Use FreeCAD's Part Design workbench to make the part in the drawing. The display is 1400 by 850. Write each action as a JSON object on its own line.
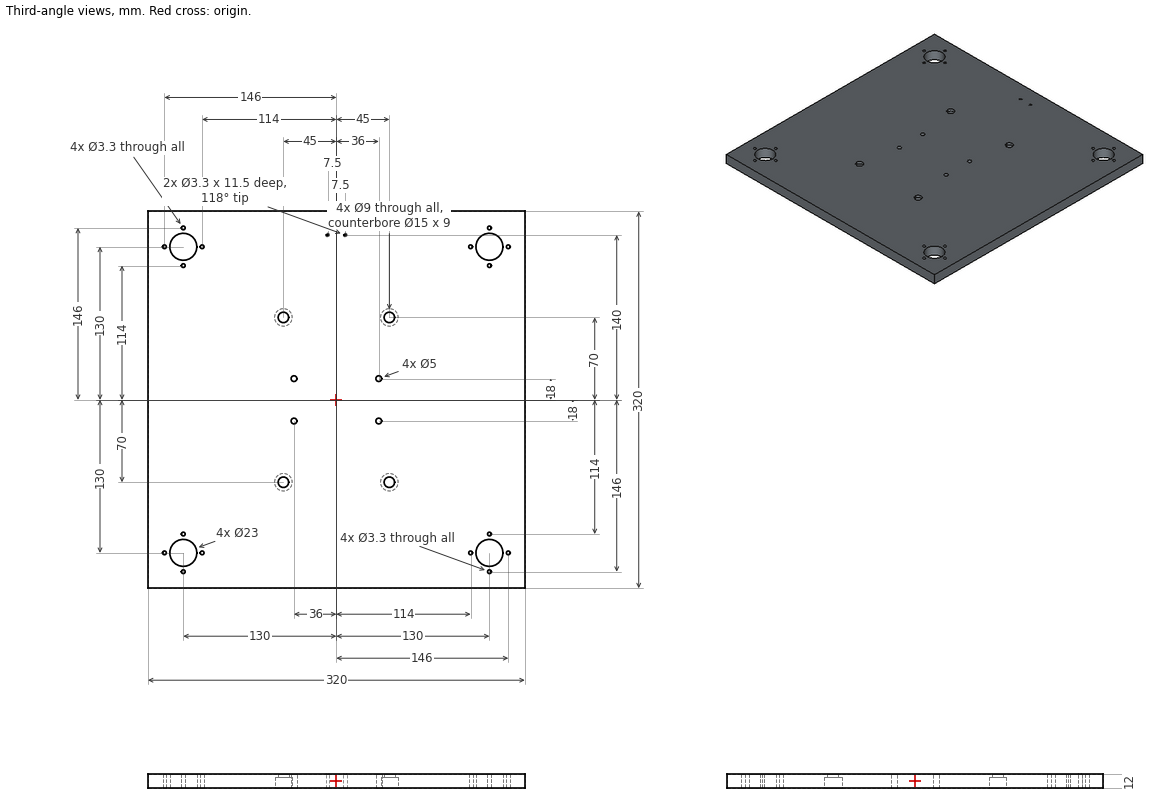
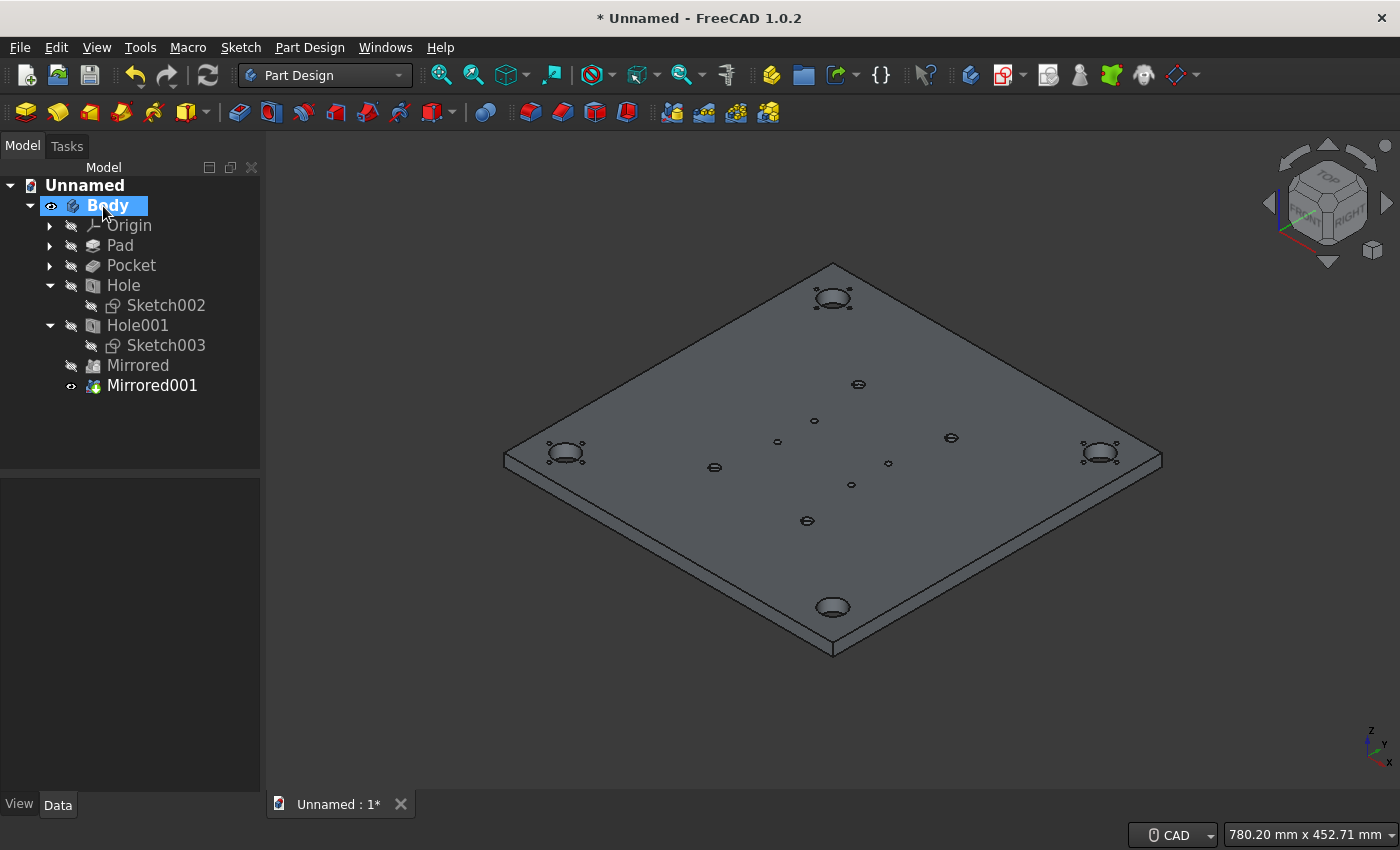
{"action": "left_click", "coordinate": [739, 398]}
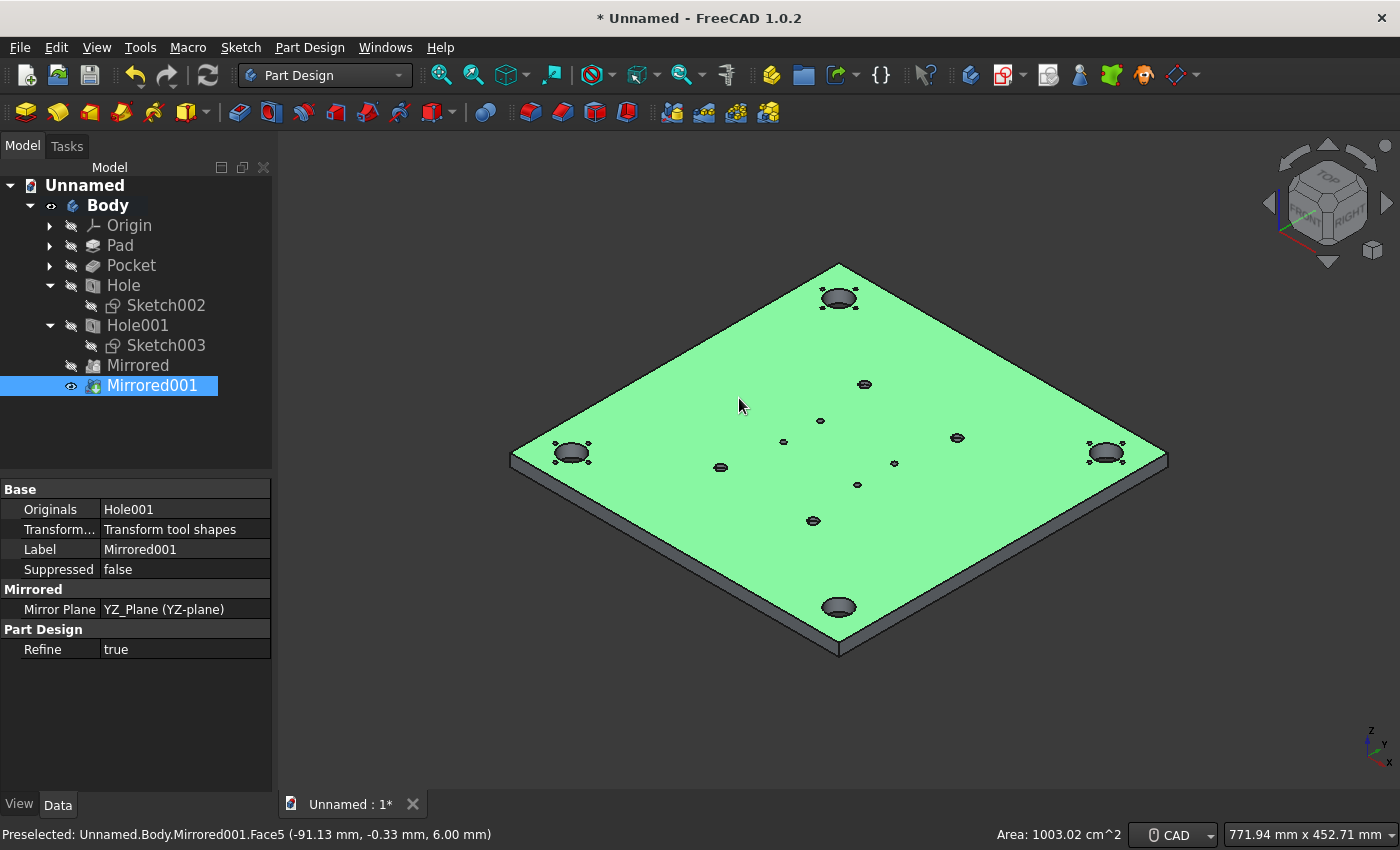
{"action": "left_click", "coordinate": [1004, 76]}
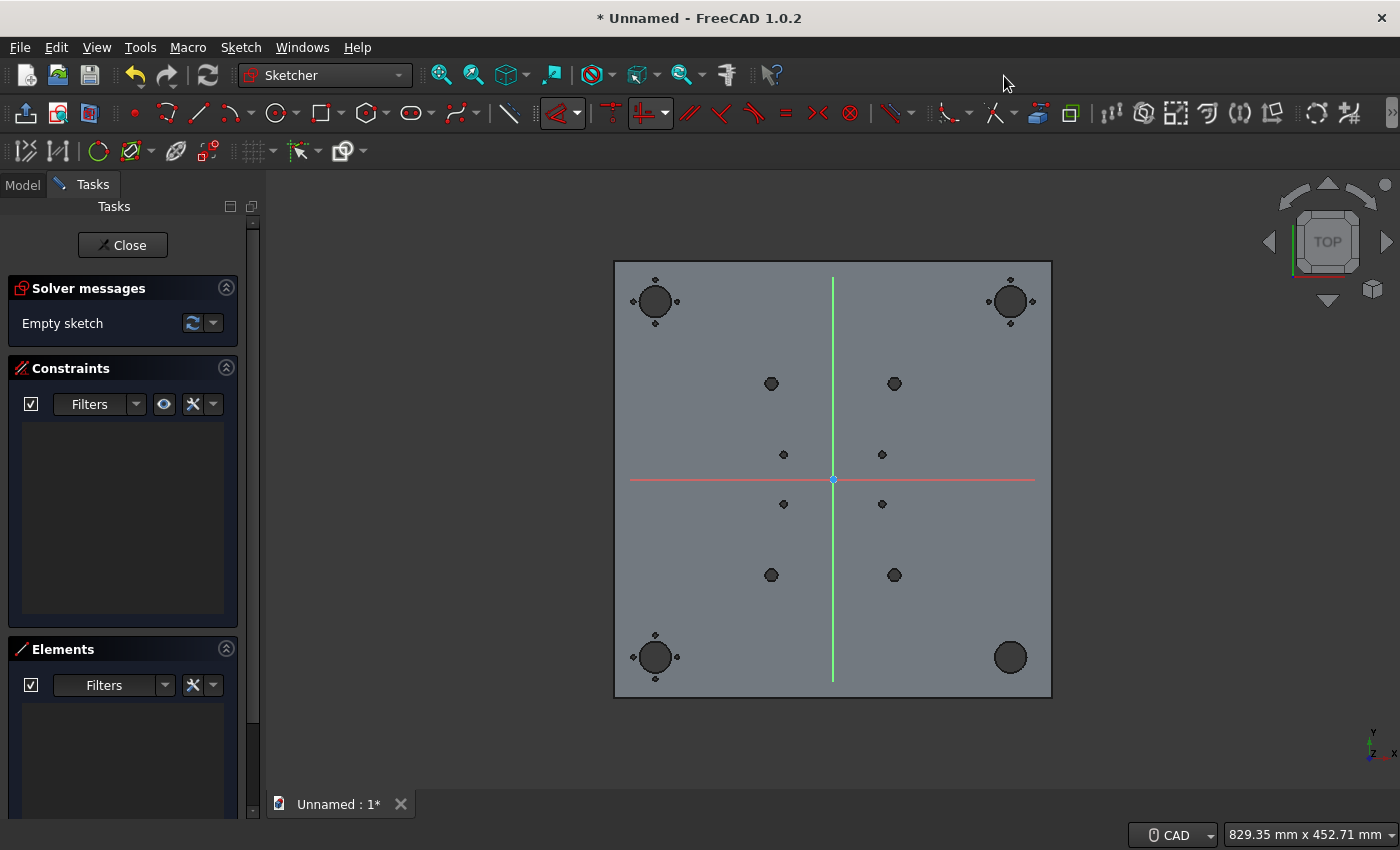
{"action": "scroll", "coordinate": [1041, 679], "scroll_direction": "up", "scroll_amount": 11}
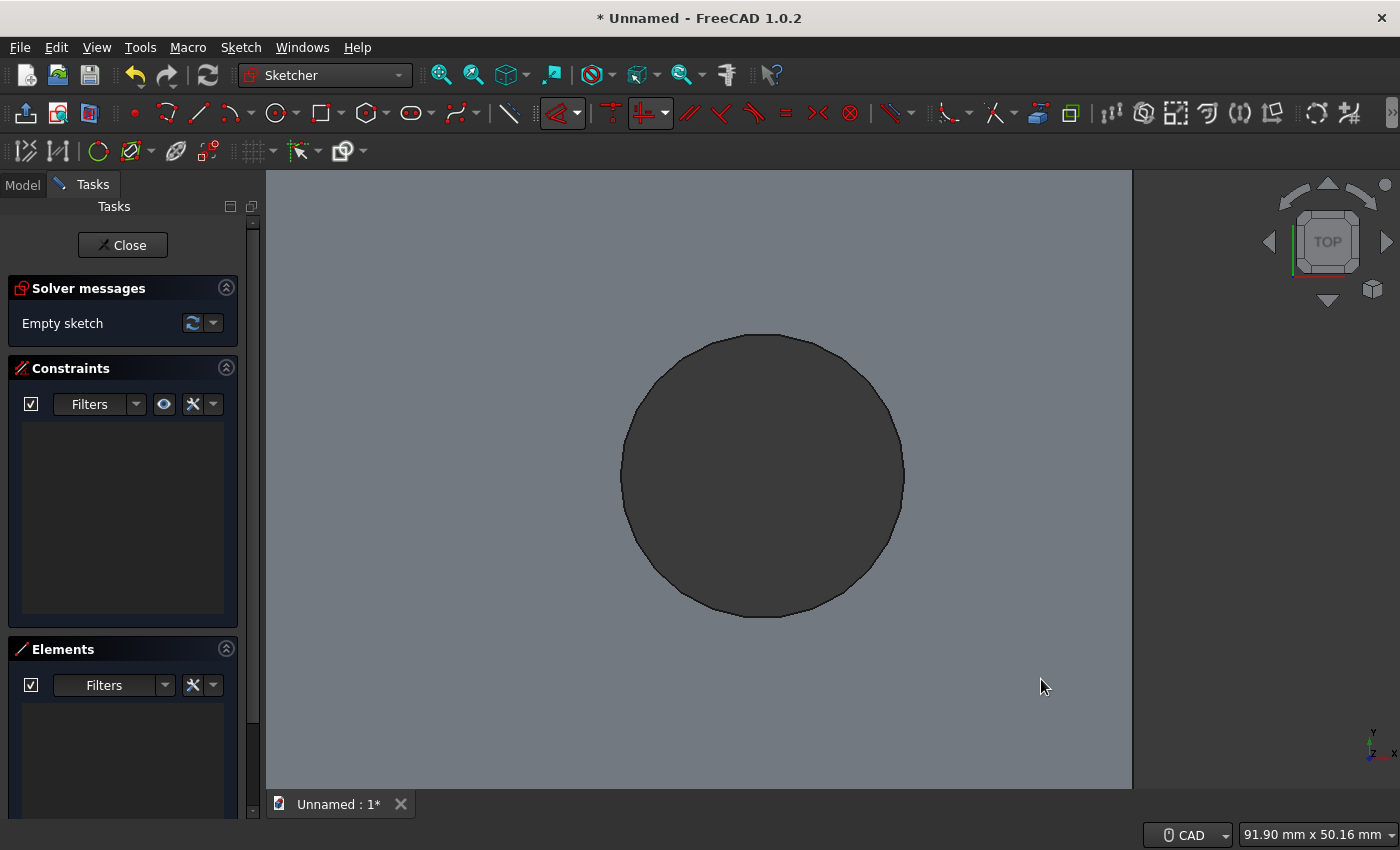
{"action": "left_click", "coordinate": [276, 114]}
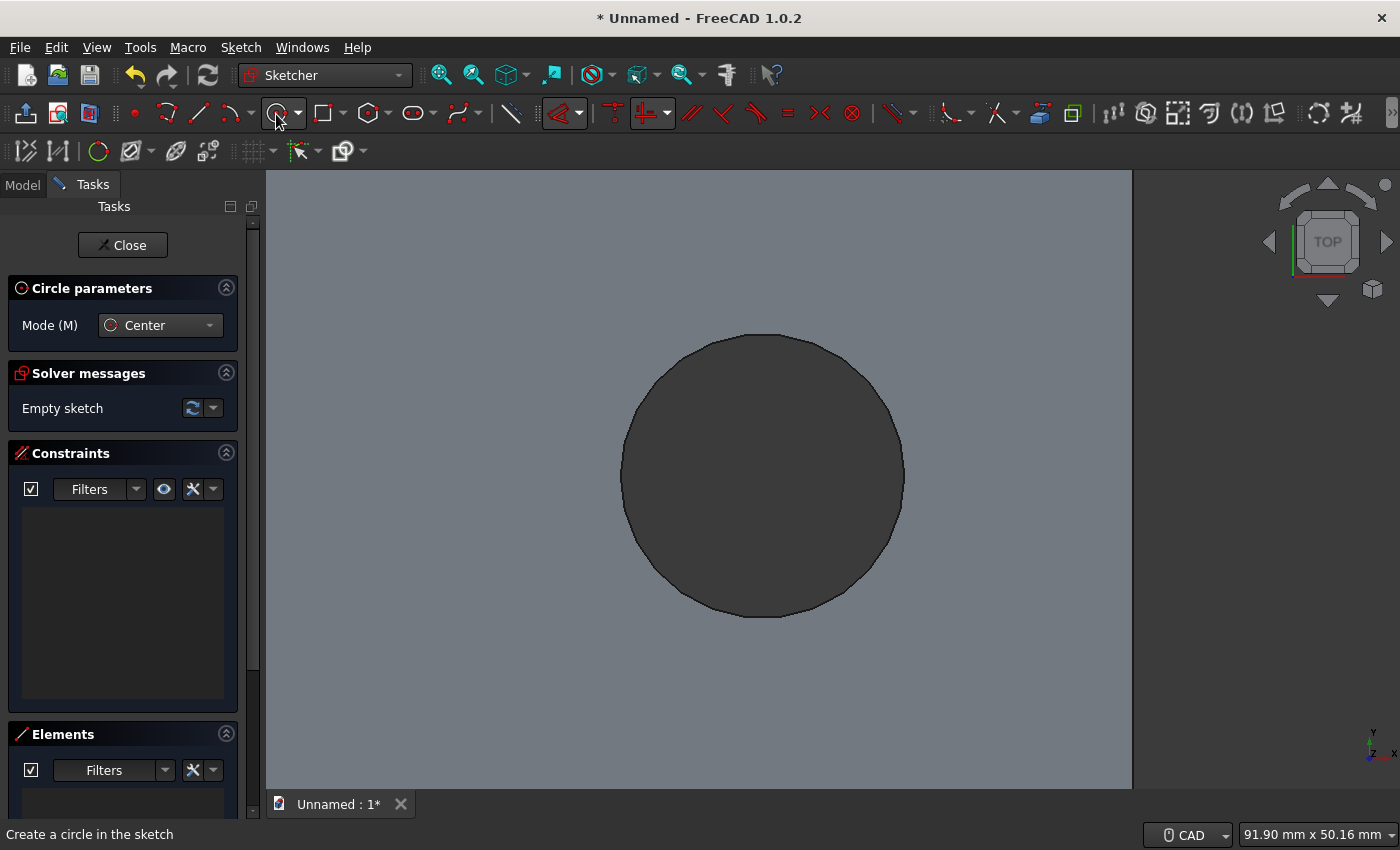
{"action": "left_click", "coordinate": [763, 674]}
{"action": "mouse_move", "coordinate": [777, 659]}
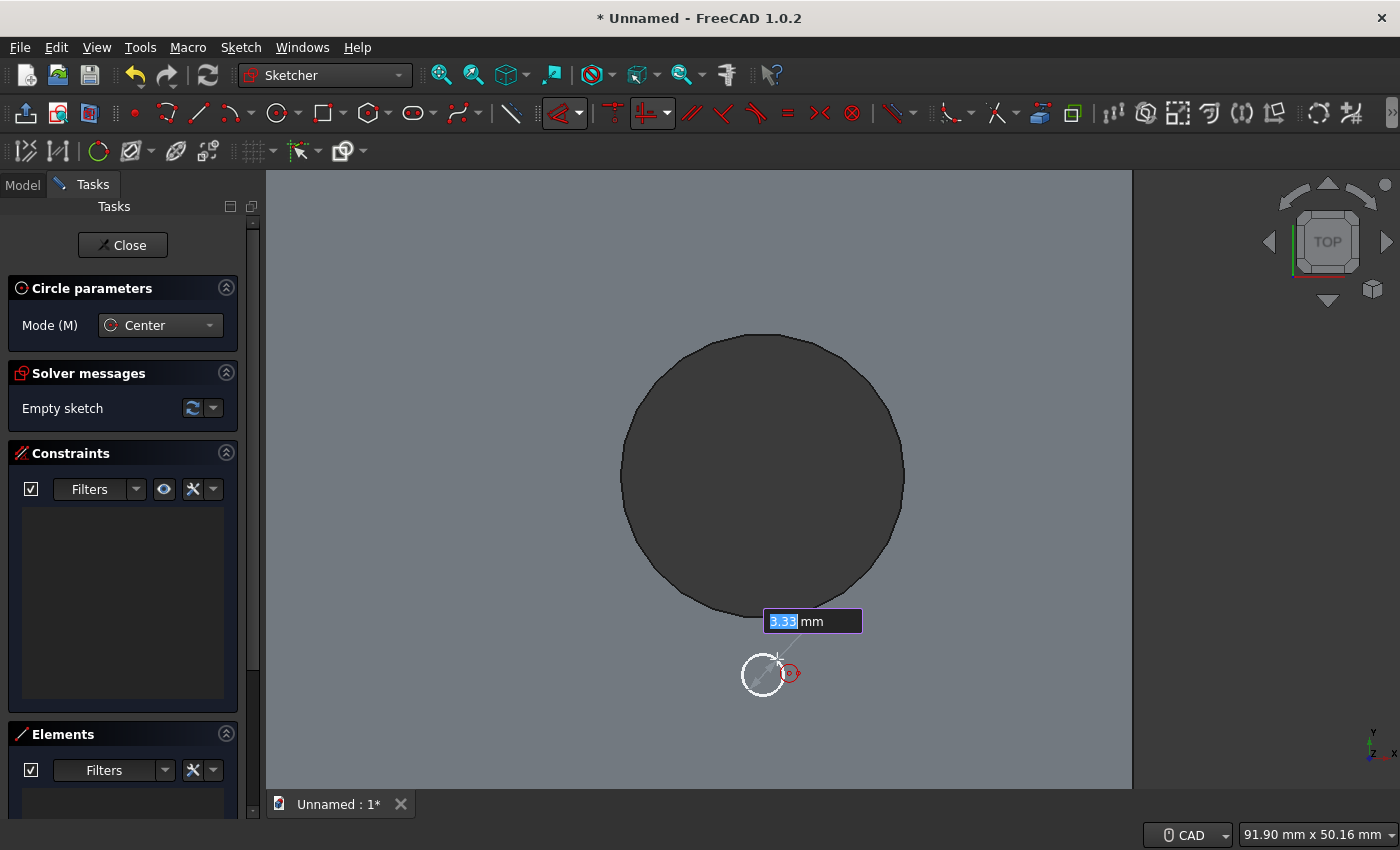
{"action": "type", "text": "3.3"}
{"action": "key", "text": "Return"}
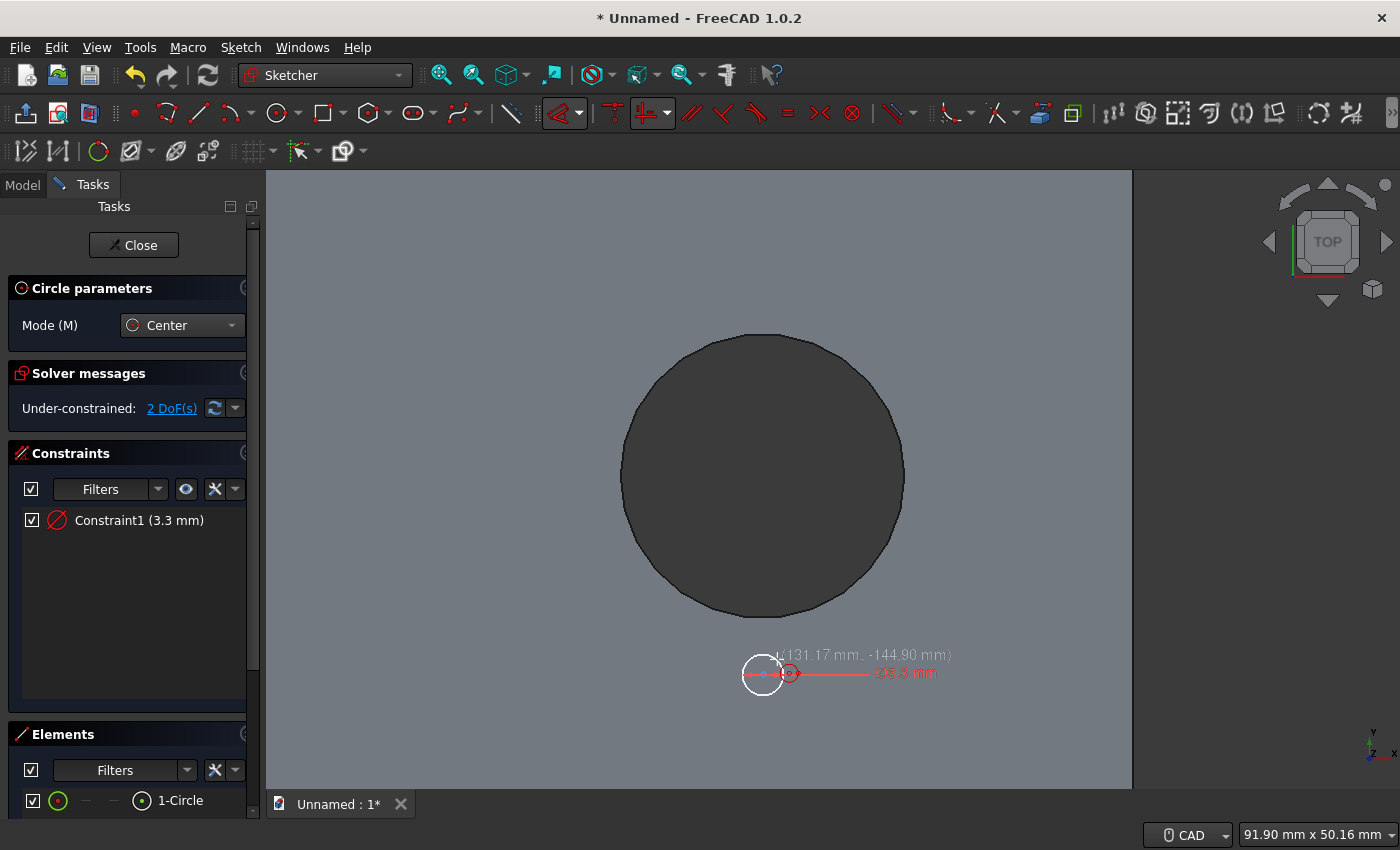
{"action": "left_click", "coordinate": [565, 476]}
{"action": "mouse_move", "coordinate": [579, 462]}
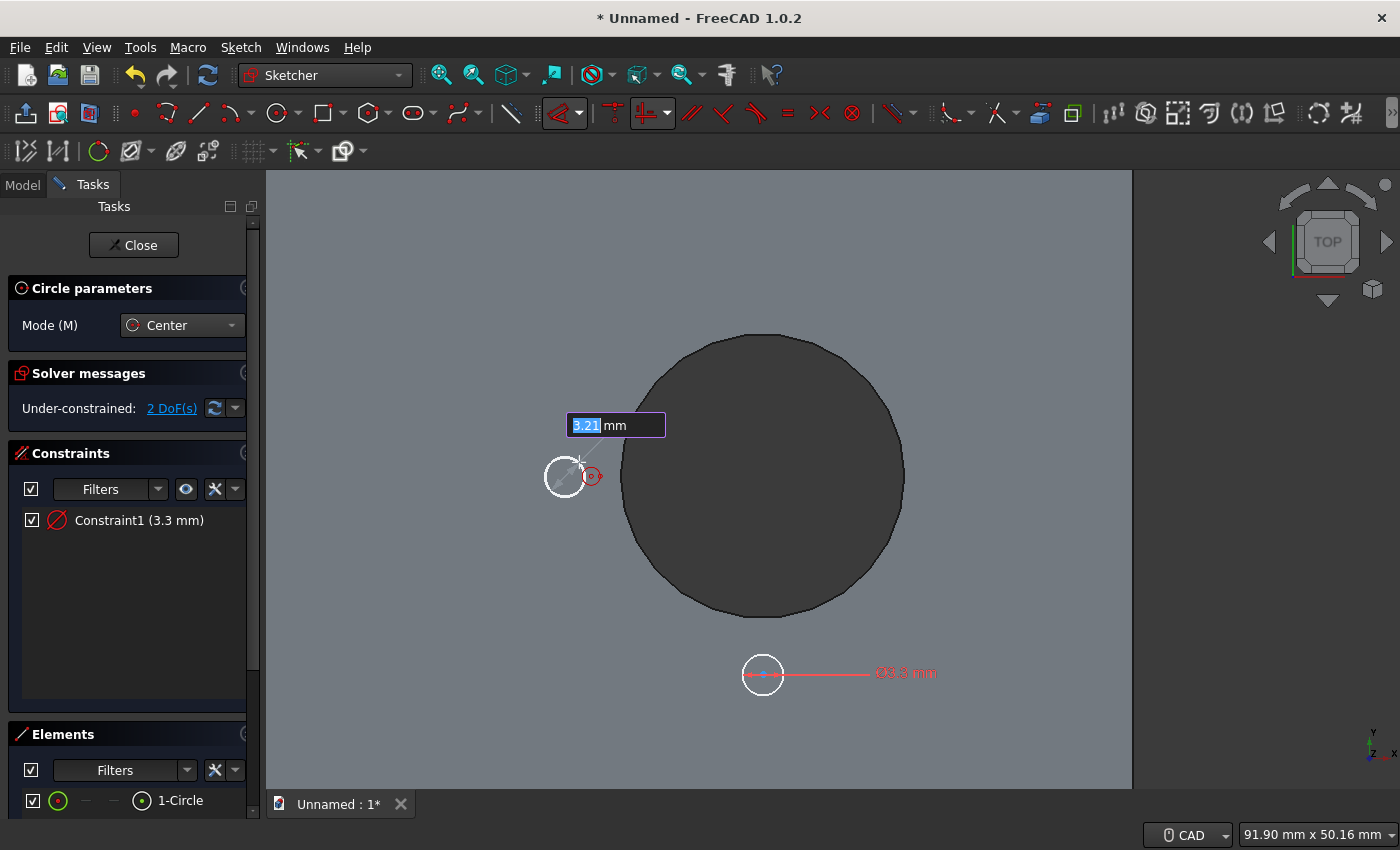
{"action": "type", "text": "3.3"}
{"action": "key", "text": "Return"}